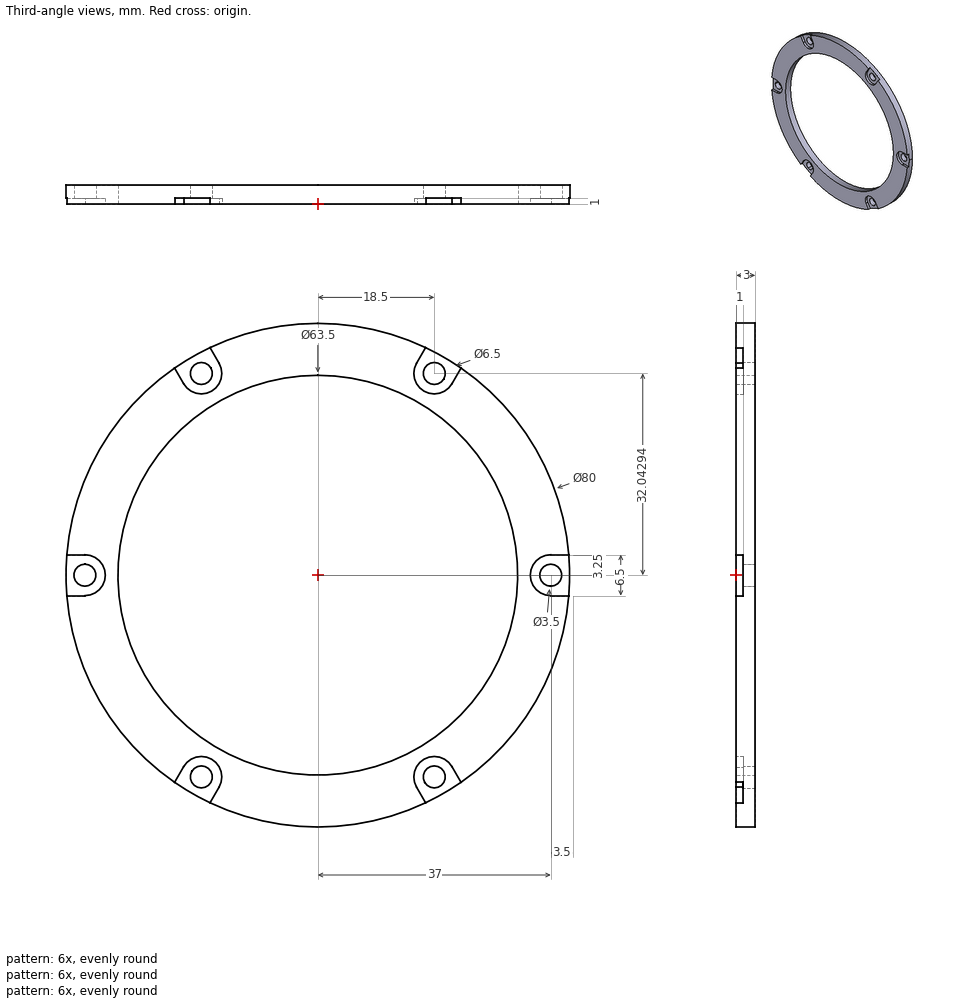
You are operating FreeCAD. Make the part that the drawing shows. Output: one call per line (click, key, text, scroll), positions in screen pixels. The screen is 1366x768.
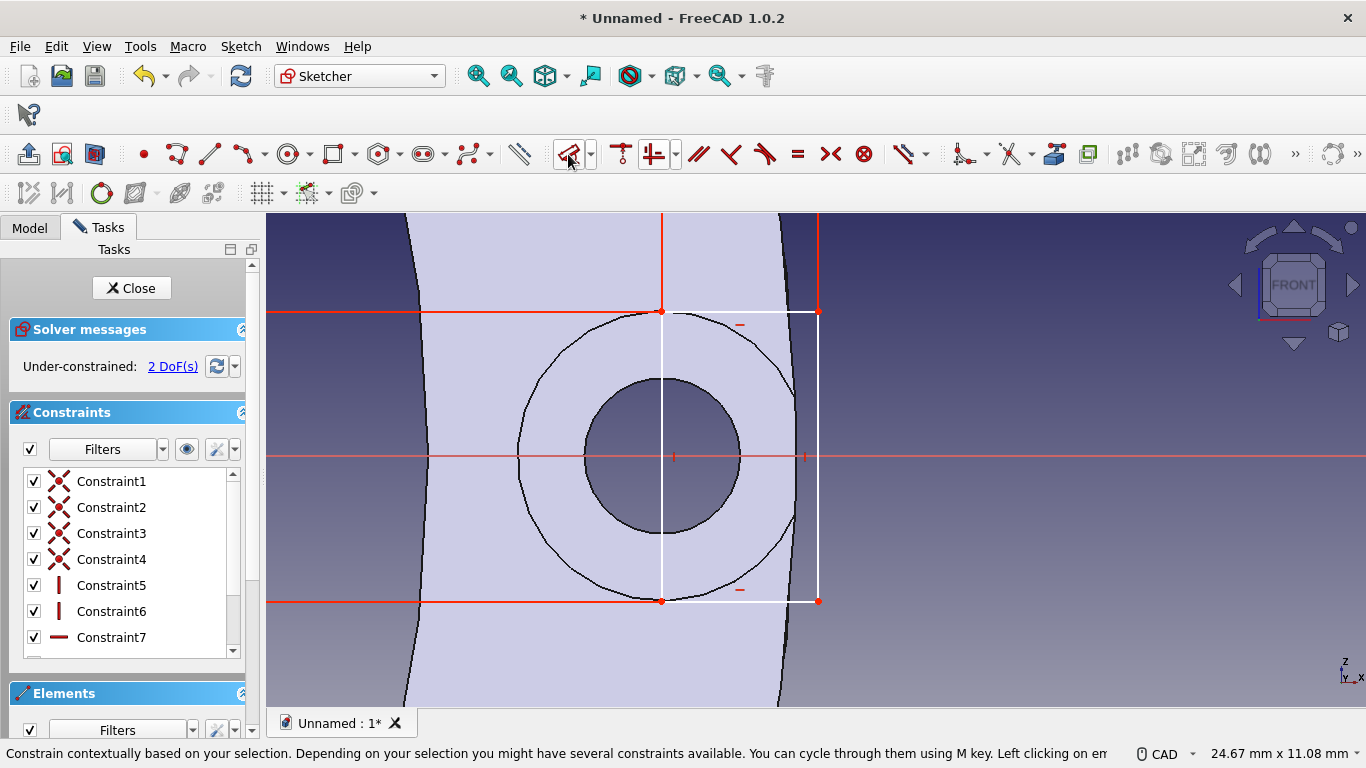
click(662, 312)
click(478, 278)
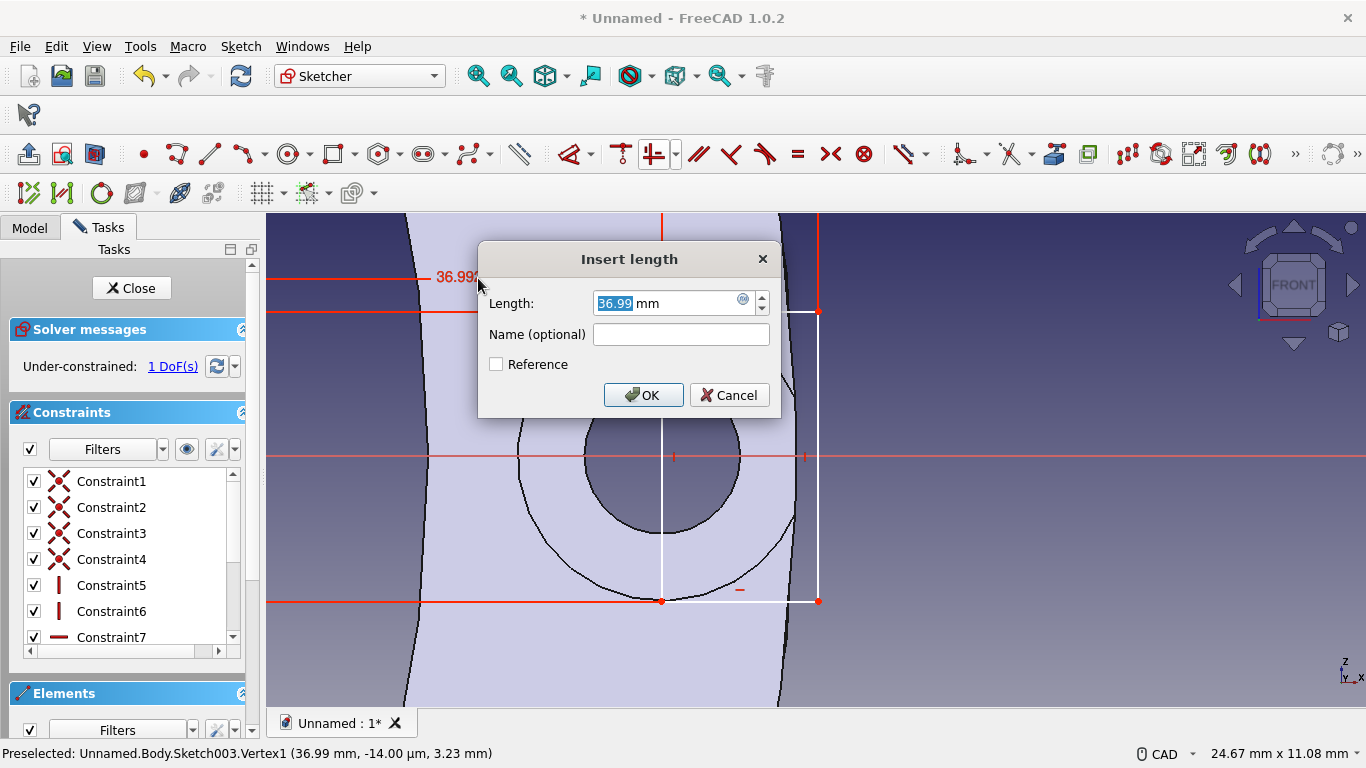
text(37)
key(Return)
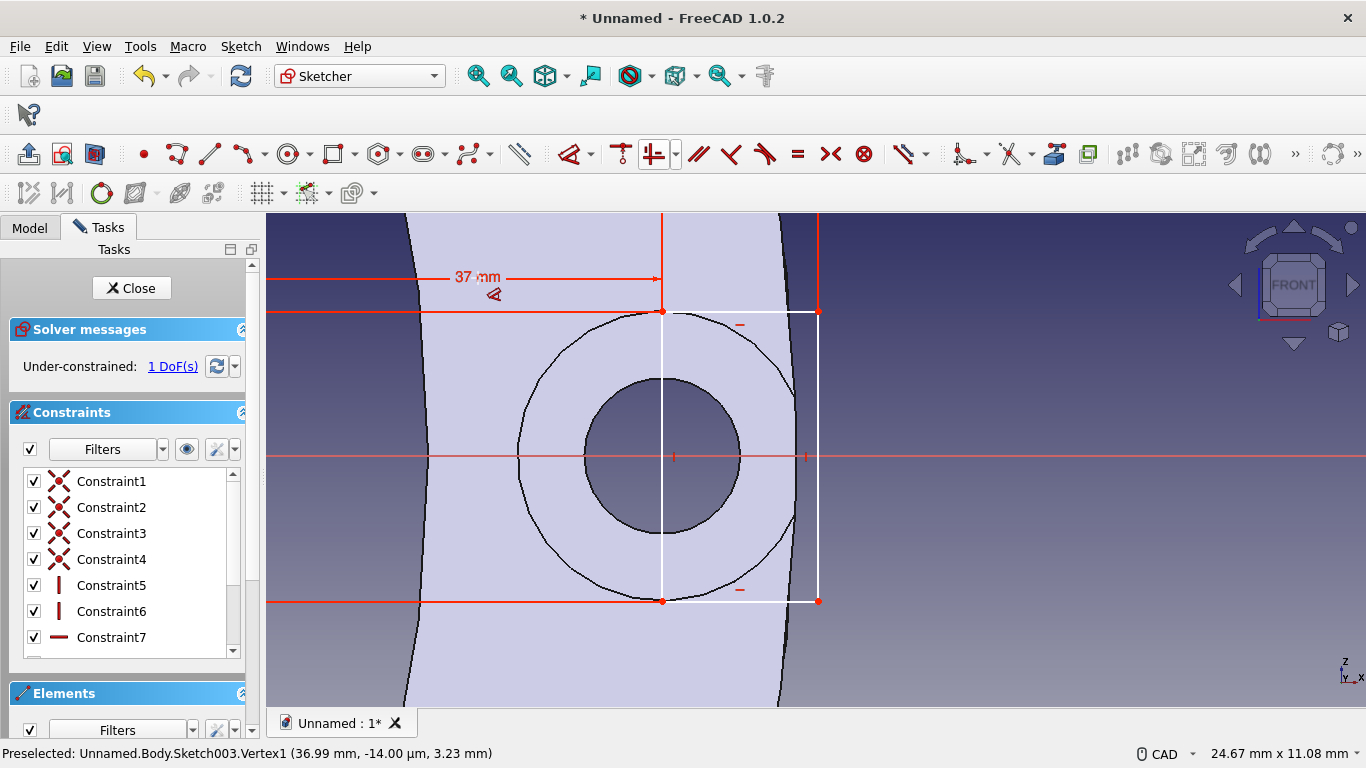
click(662, 312)
click(696, 384)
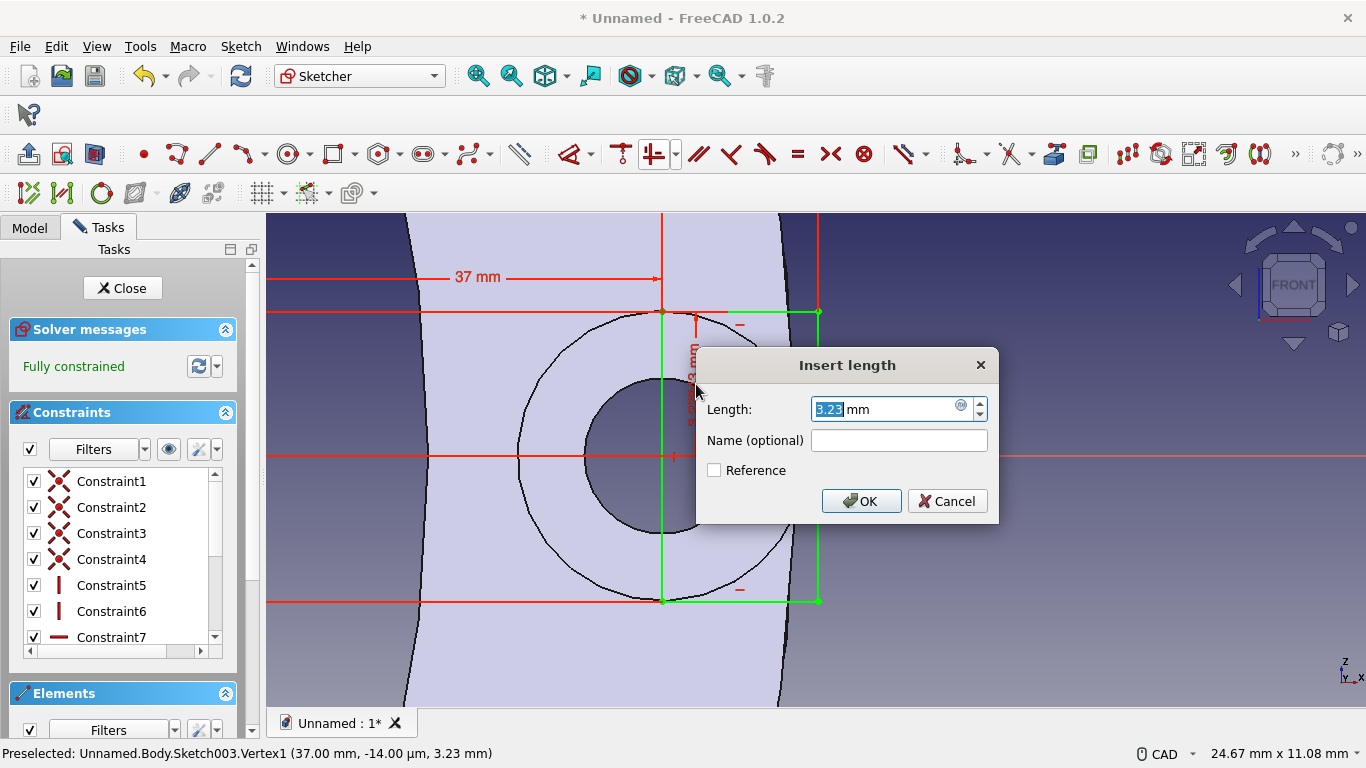
text(3.25)
key(Return)
key(Escape)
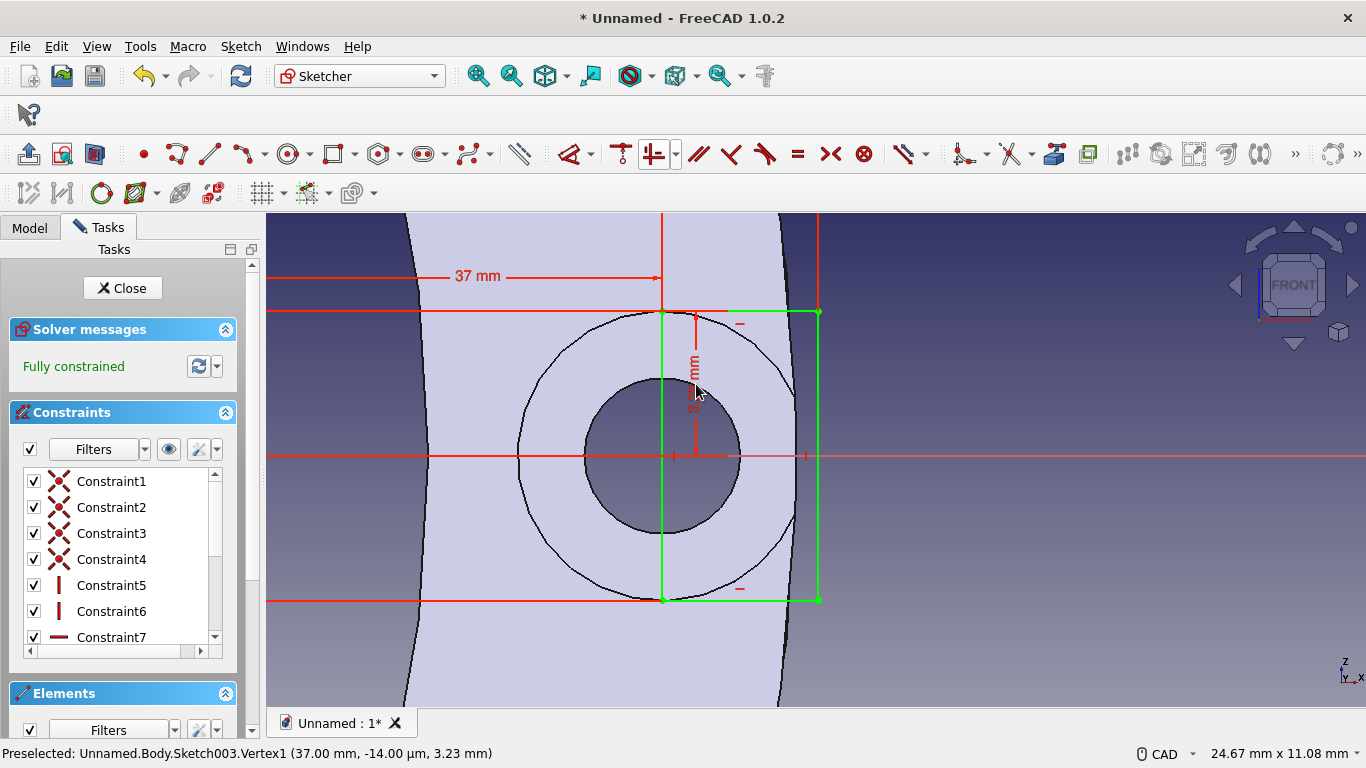
click(123, 288)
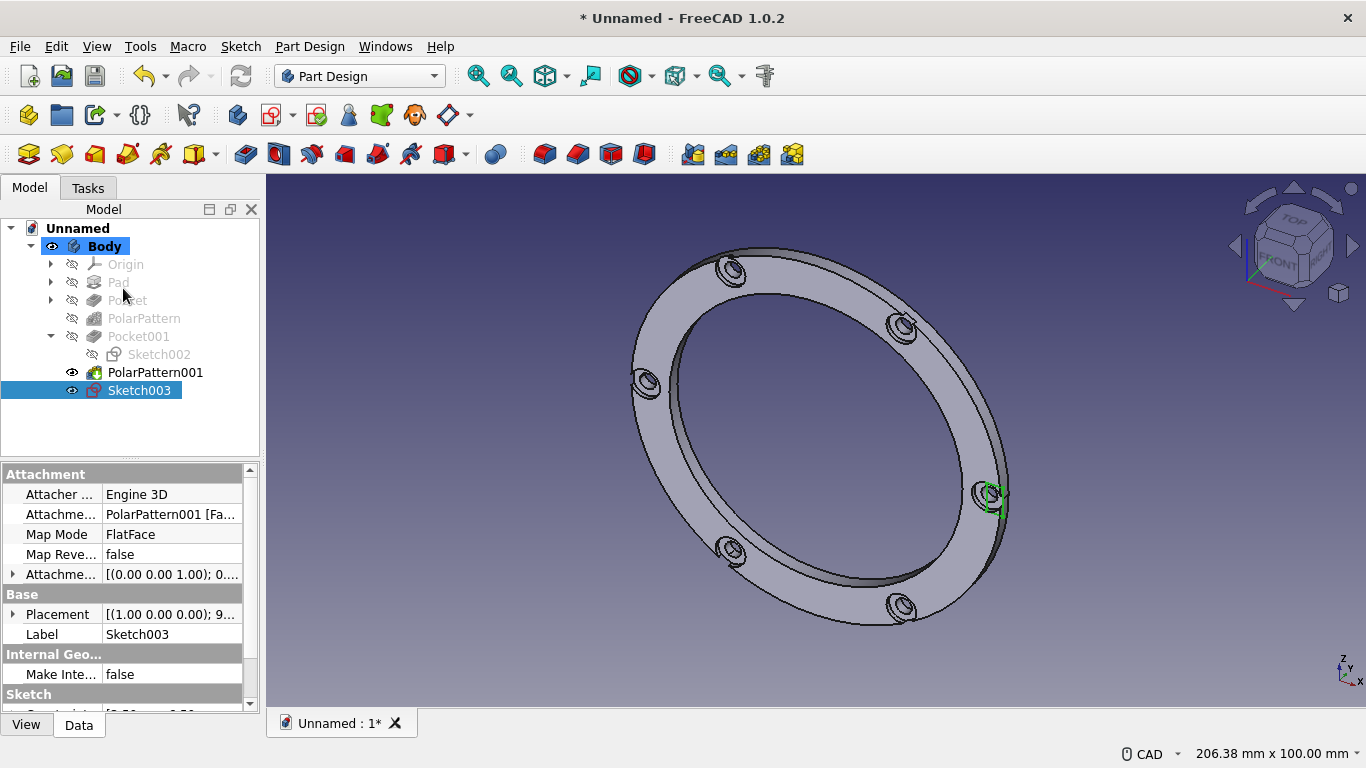
click(246, 154)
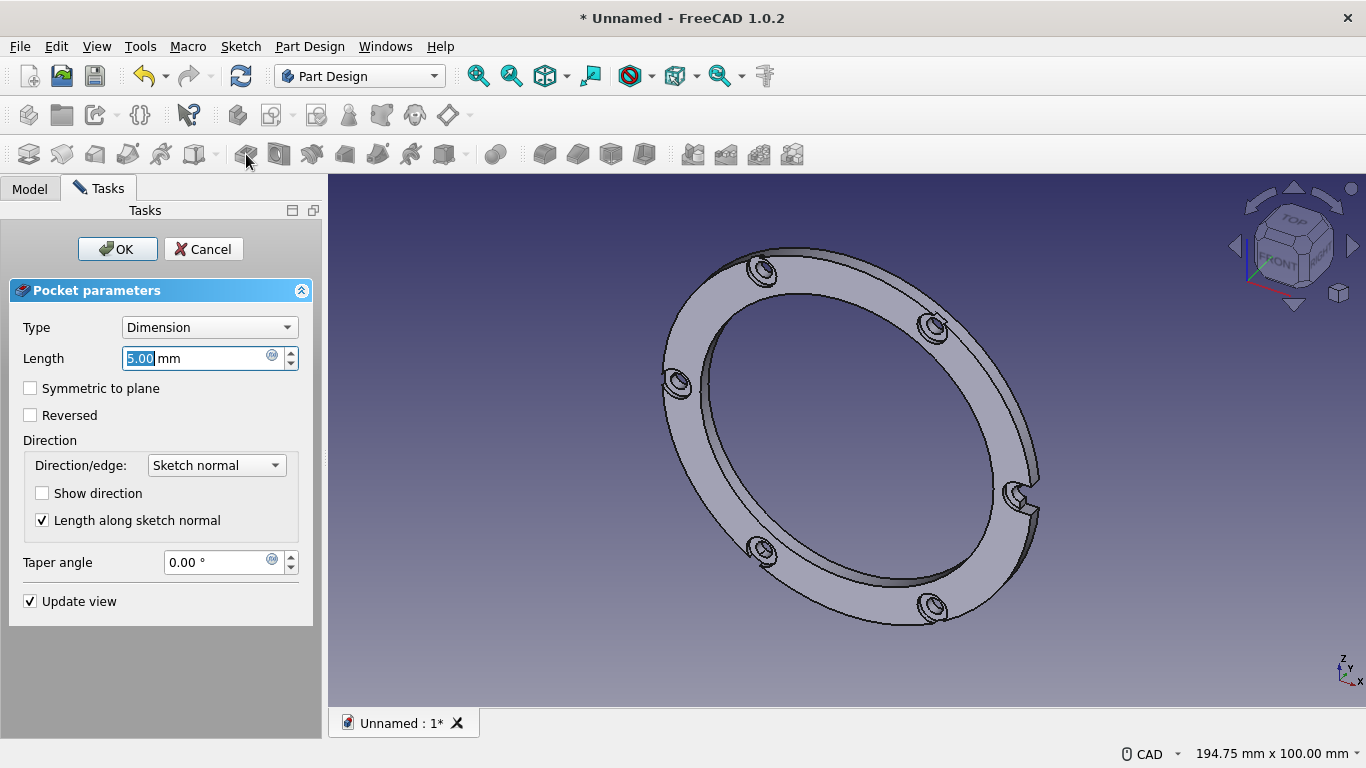
text(1)
key(Tab)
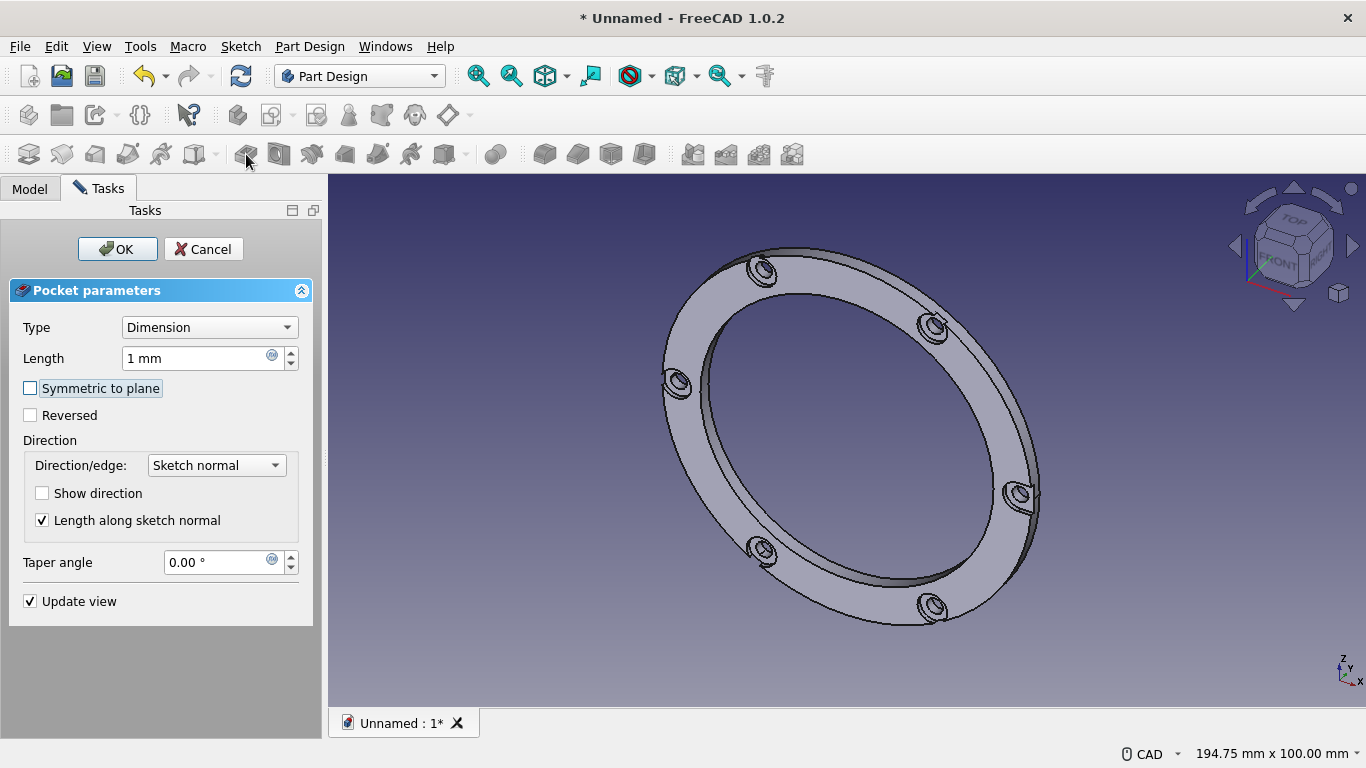
click(118, 249)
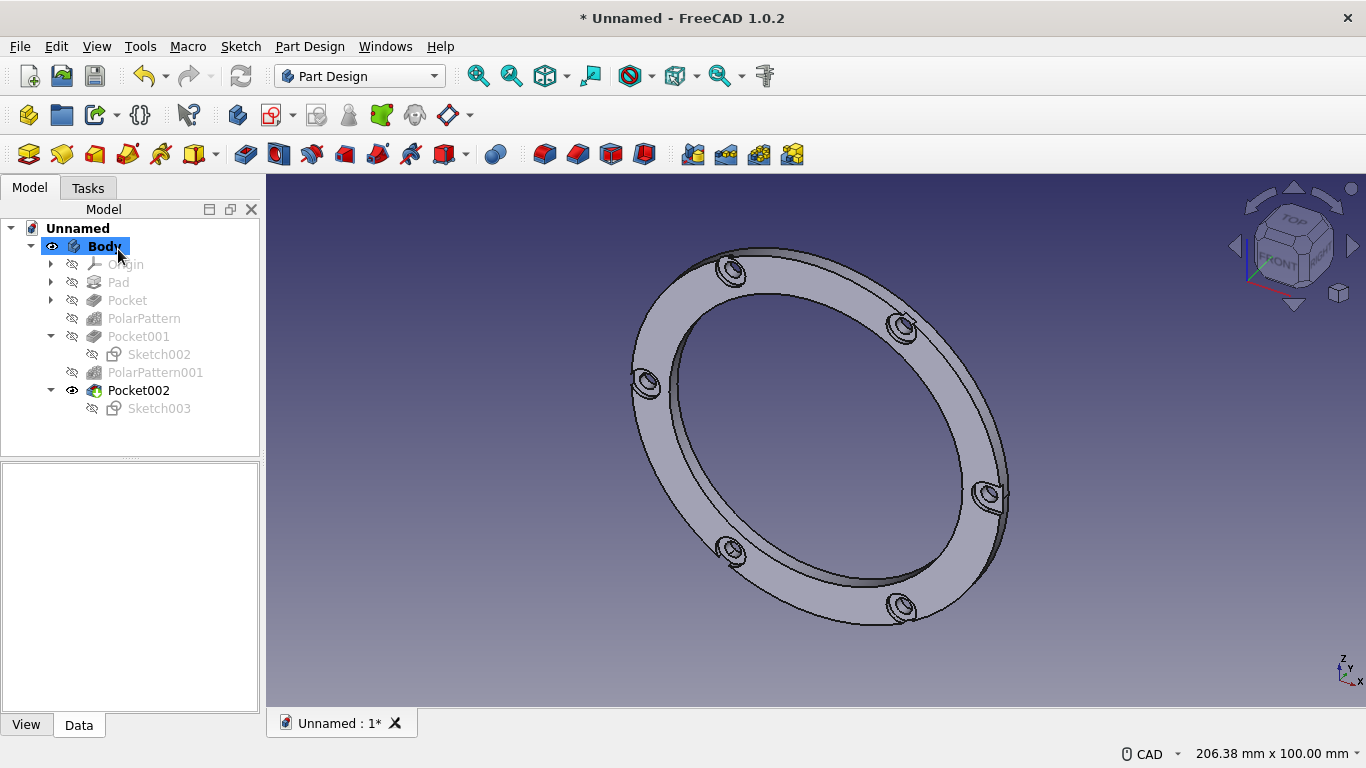
click(117, 390)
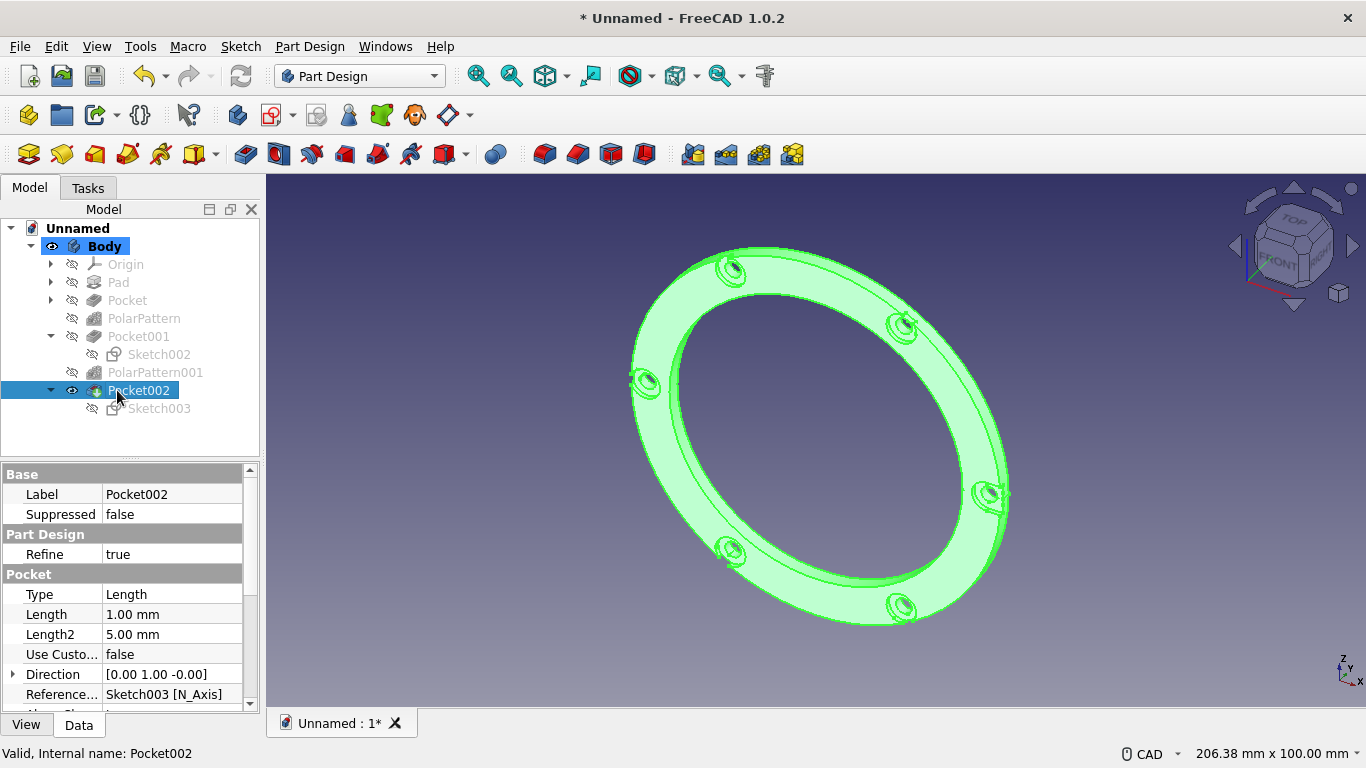
click(759, 154)